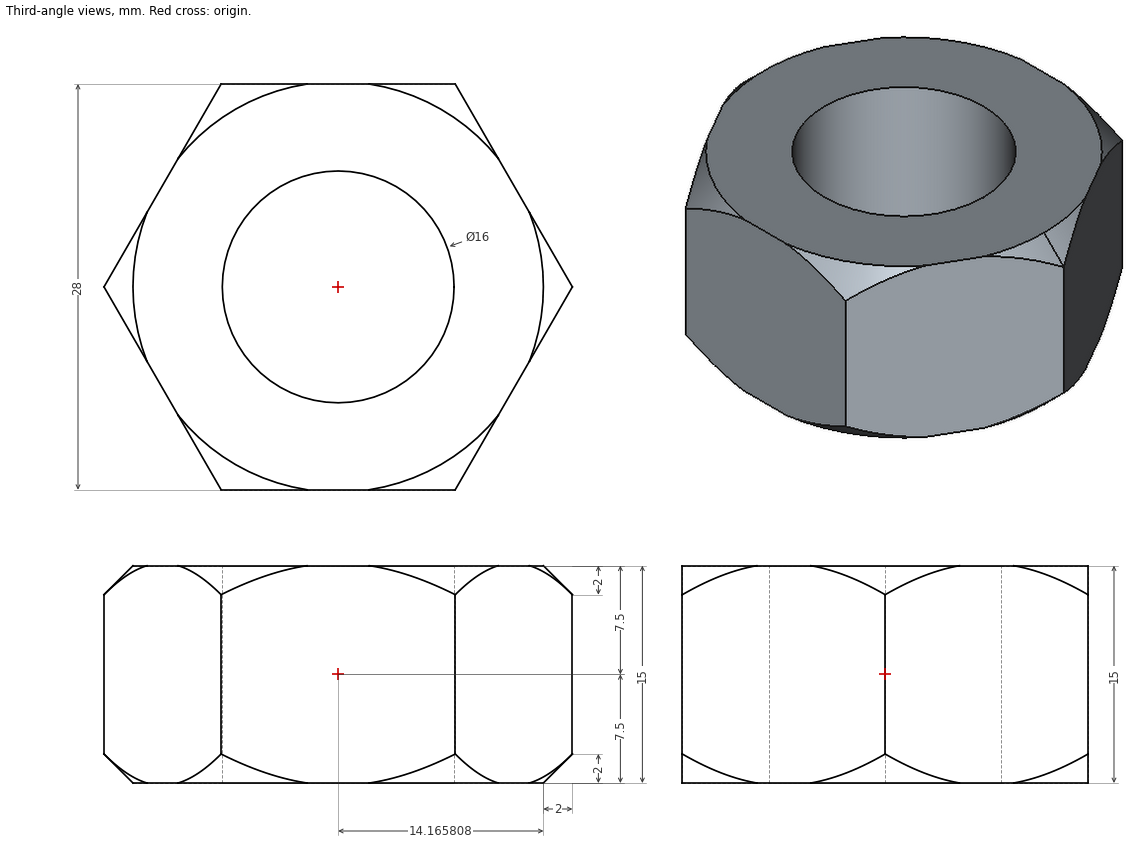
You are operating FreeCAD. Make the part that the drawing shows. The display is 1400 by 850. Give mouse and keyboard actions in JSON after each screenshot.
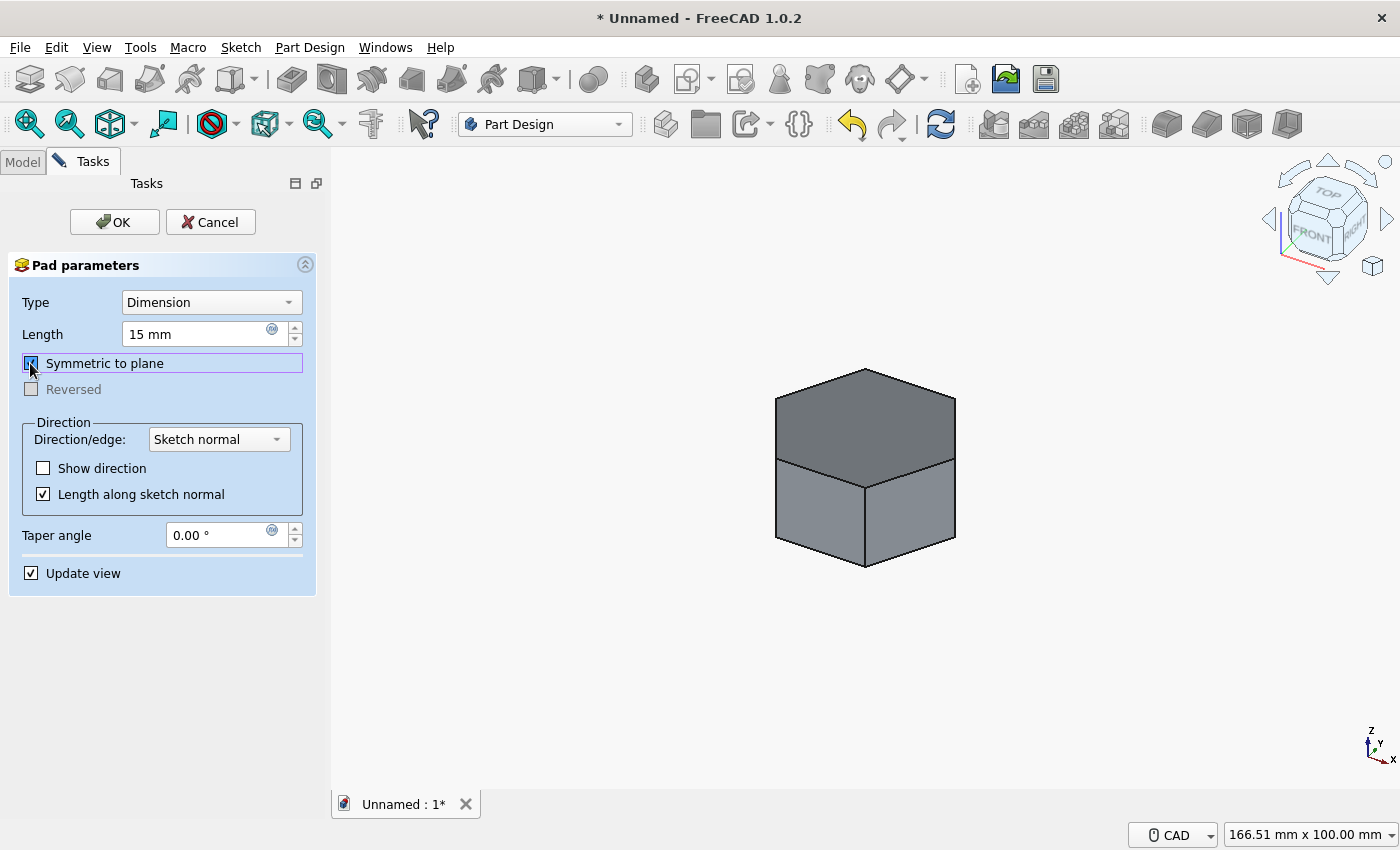
{"action": "left_click", "coordinate": [115, 222]}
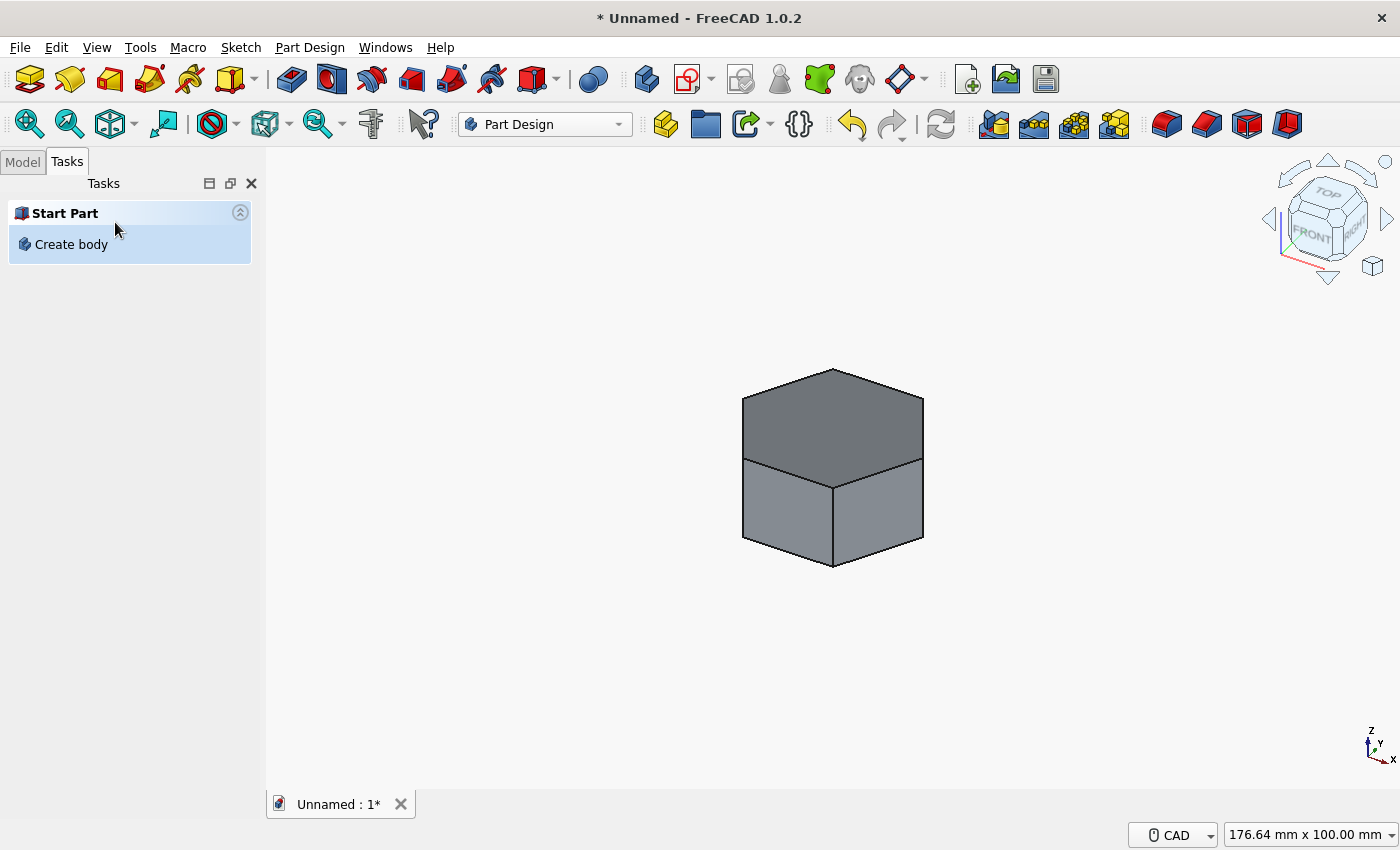
{"action": "left_click", "coordinate": [30, 124]}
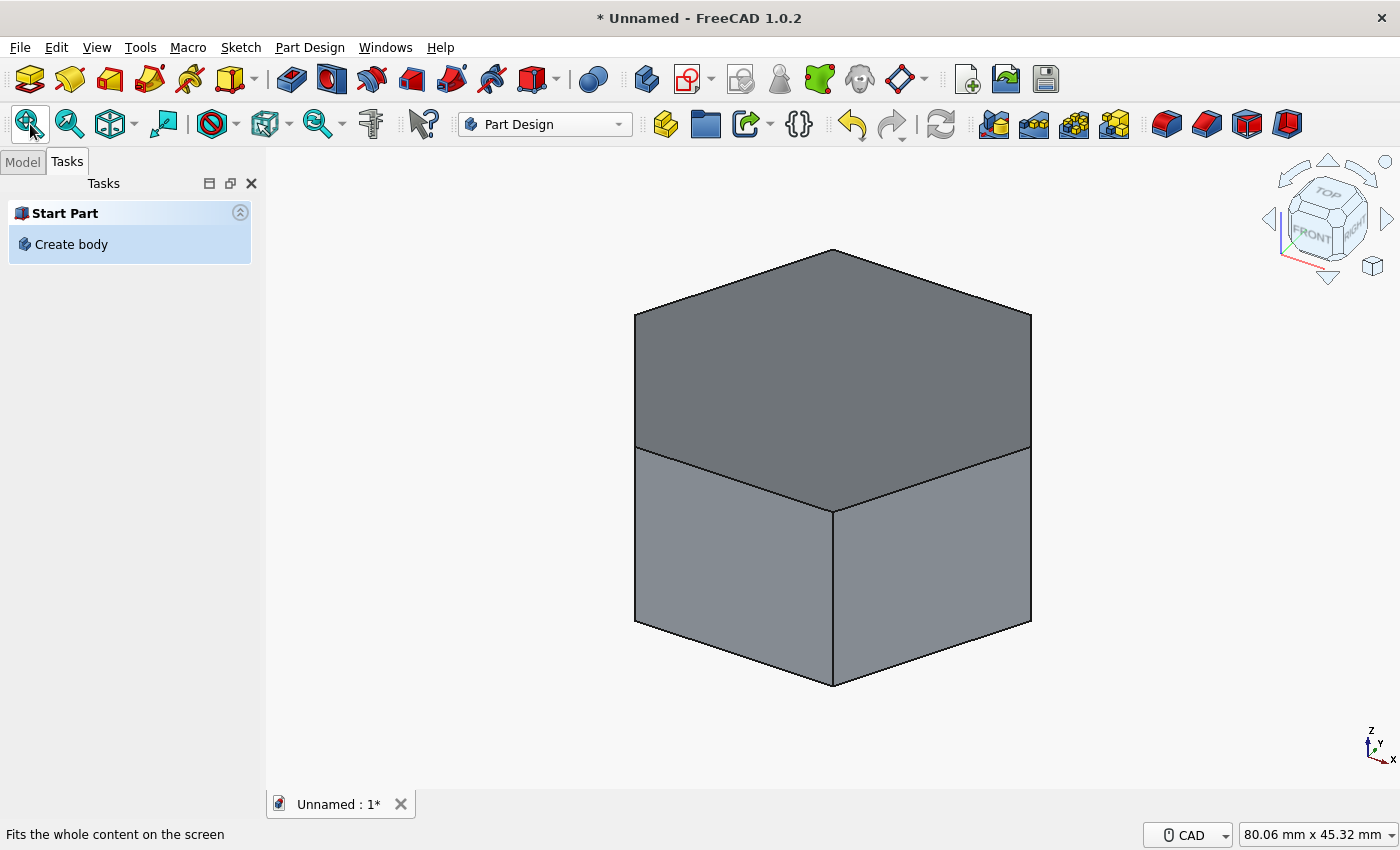
{"action": "left_click", "coordinate": [688, 80]}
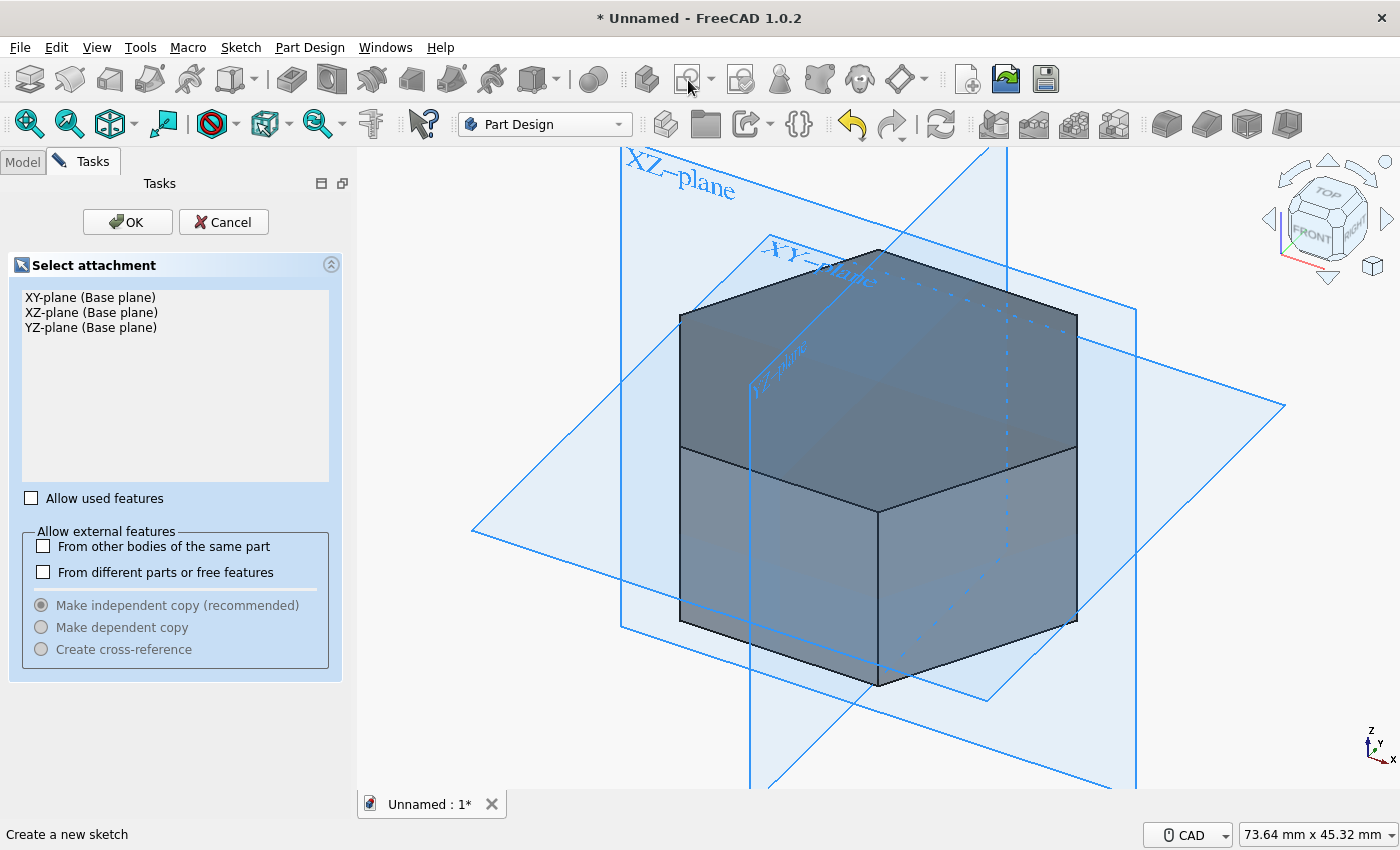
{"action": "left_click", "coordinate": [82, 298]}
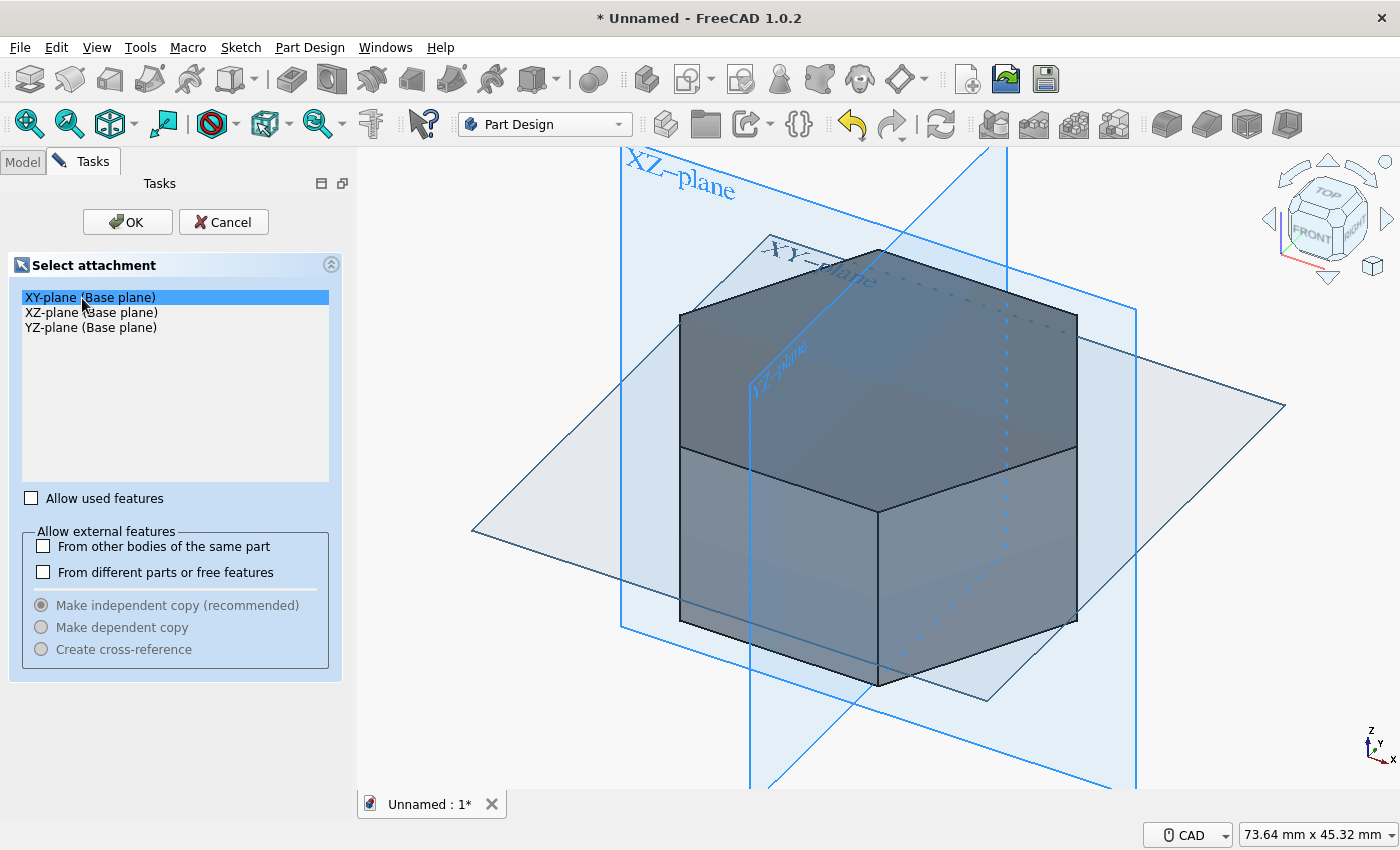
{"action": "left_click", "coordinate": [128, 222]}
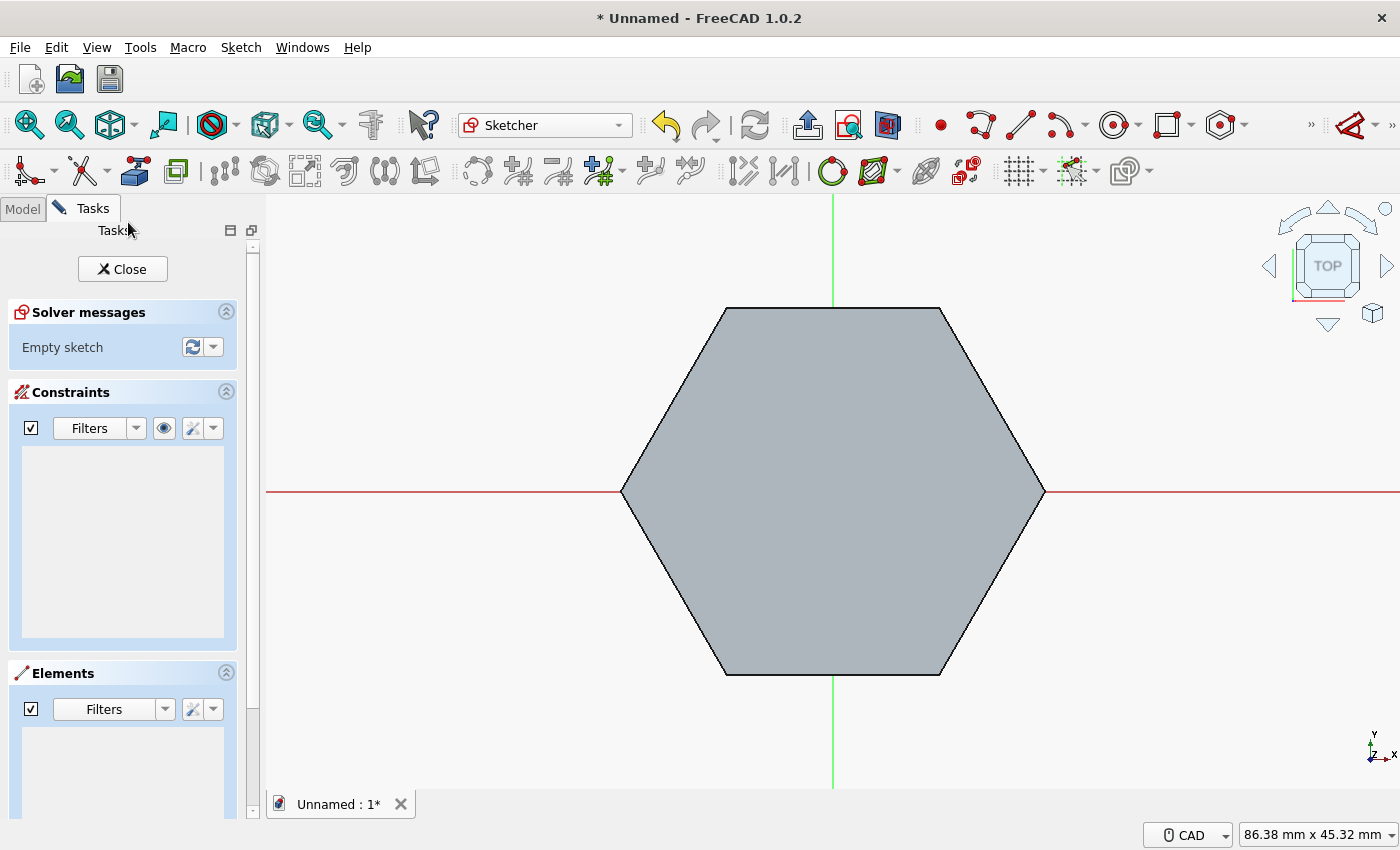
{"action": "left_click", "coordinate": [888, 126]}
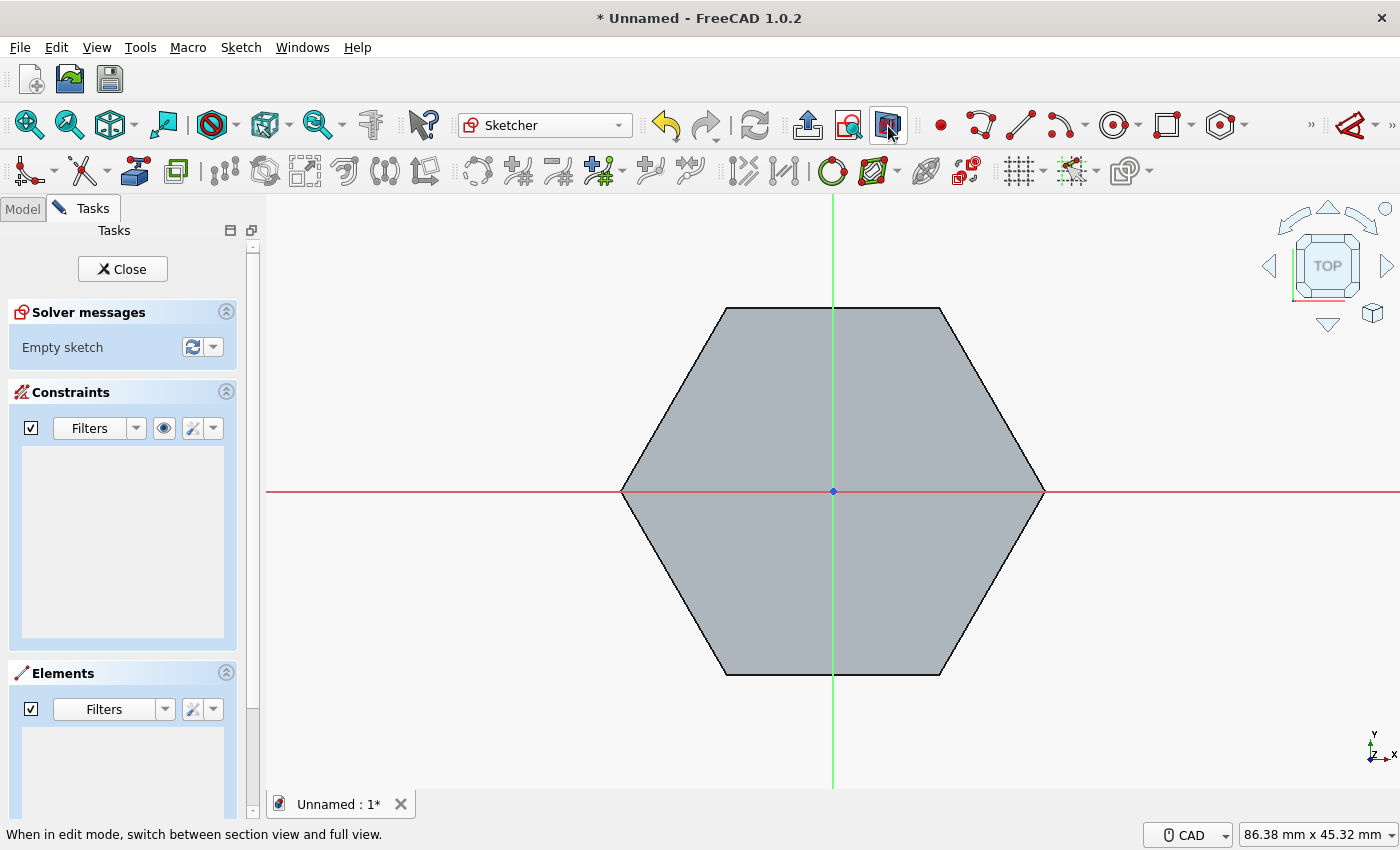
{"action": "scroll", "coordinate": [916, 492], "scroll_direction": "up", "scroll_amount": 3}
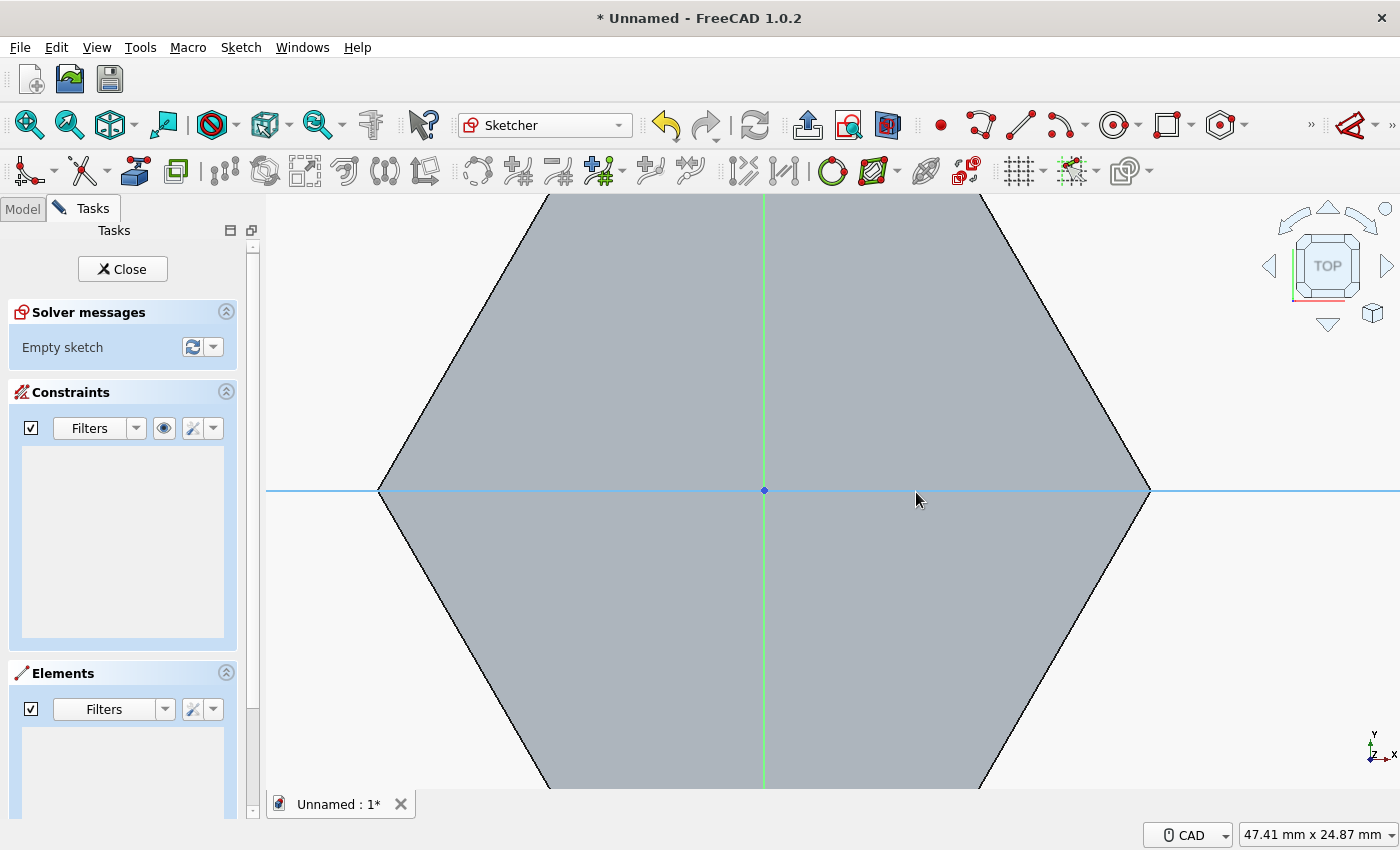
{"action": "left_click", "coordinate": [1114, 126]}